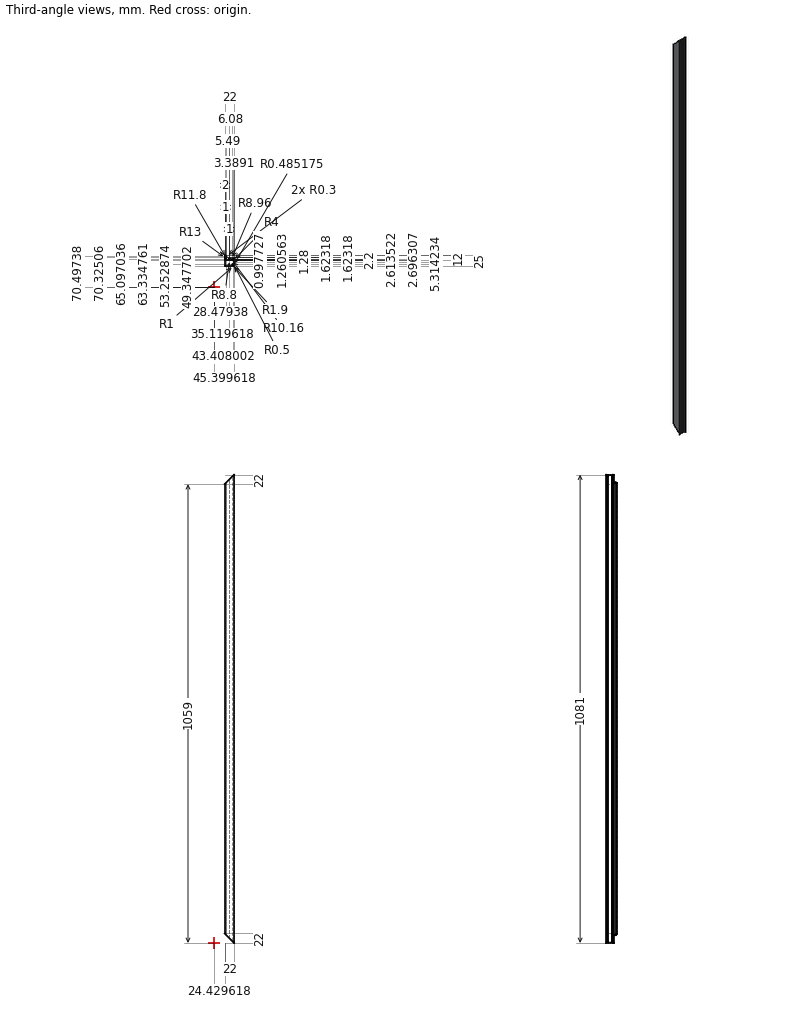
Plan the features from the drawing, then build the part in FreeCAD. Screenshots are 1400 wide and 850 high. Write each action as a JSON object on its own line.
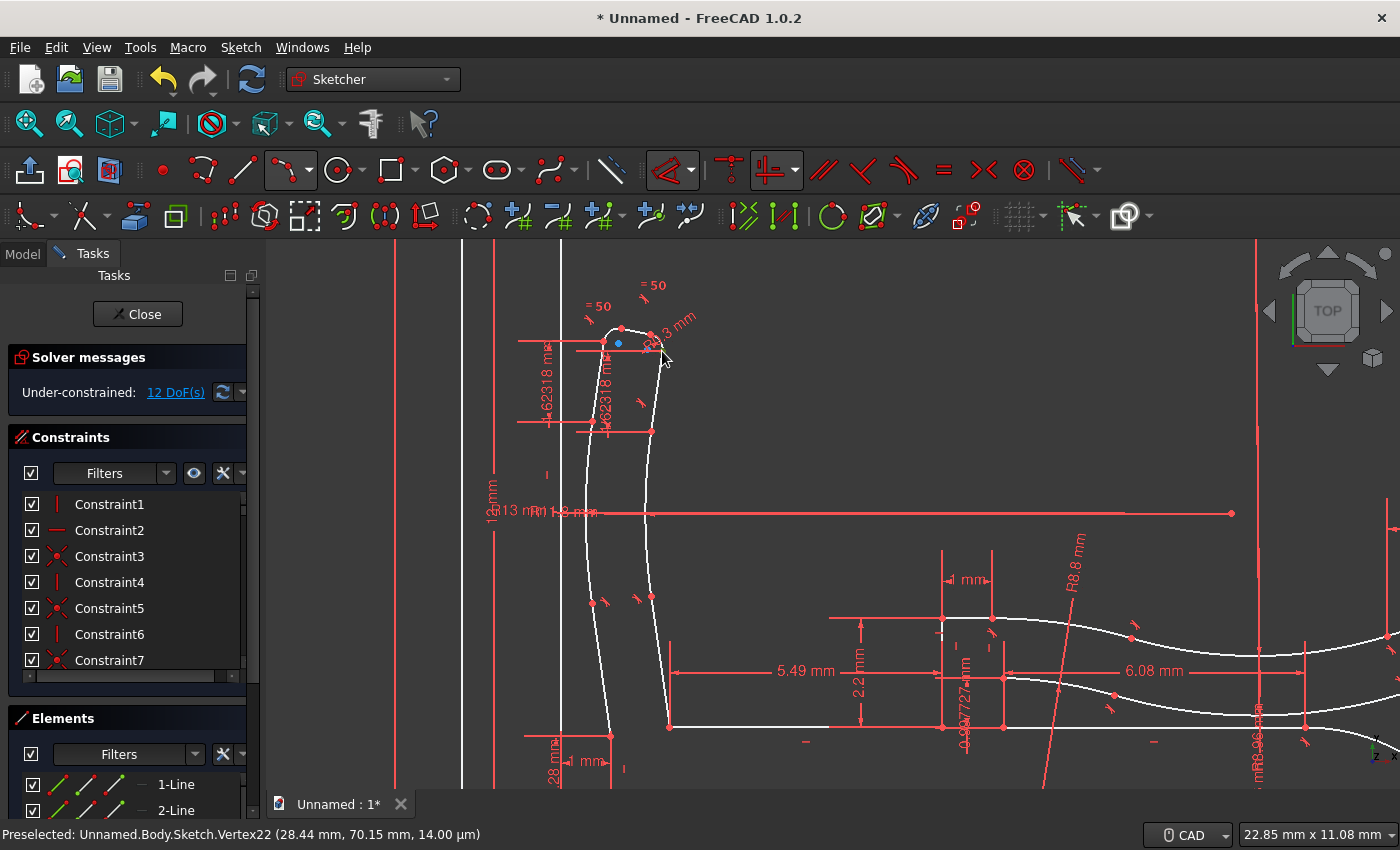
{"action": "left_click", "coordinate": [694, 170]}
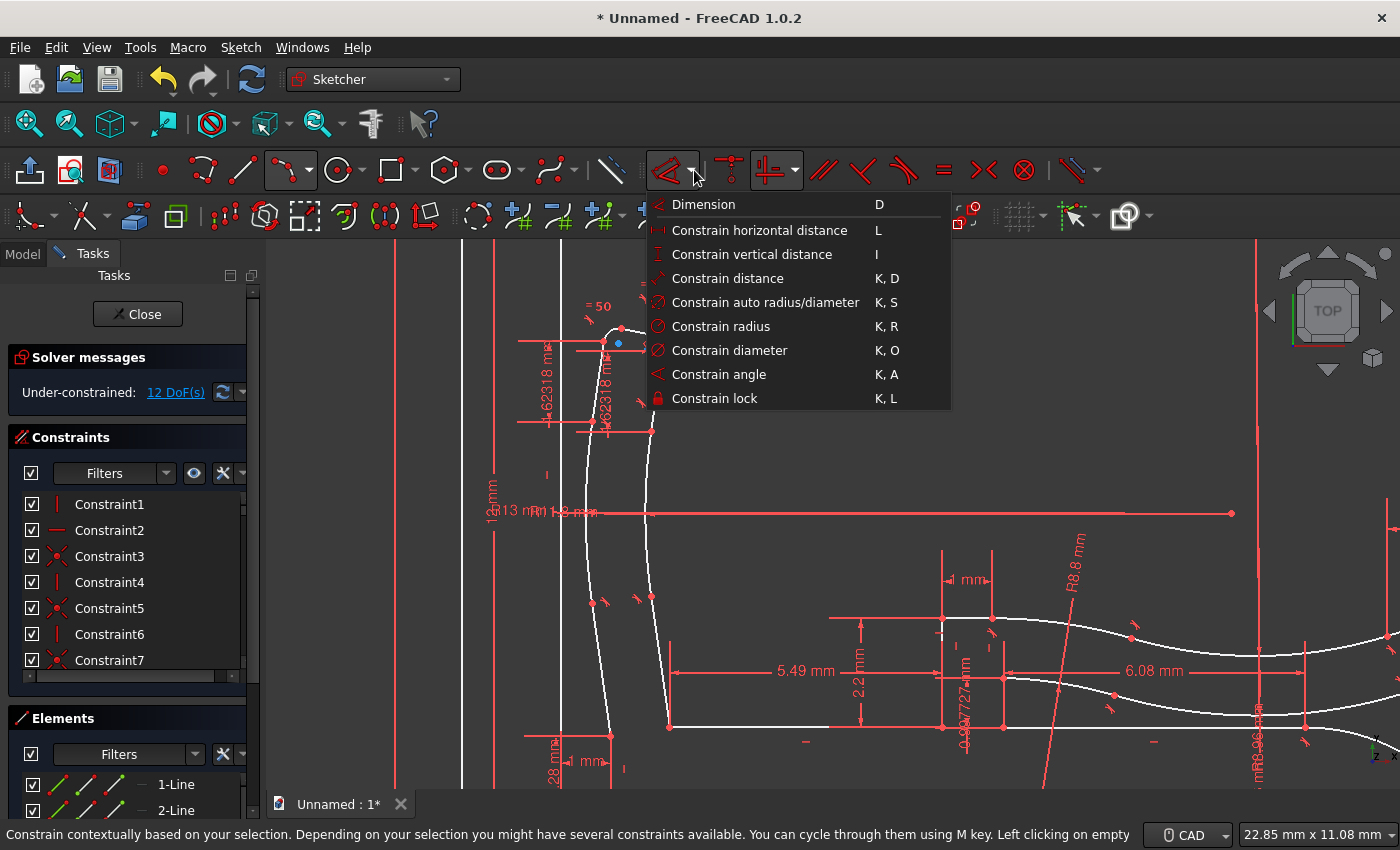
{"action": "left_click", "coordinate": [799, 230]}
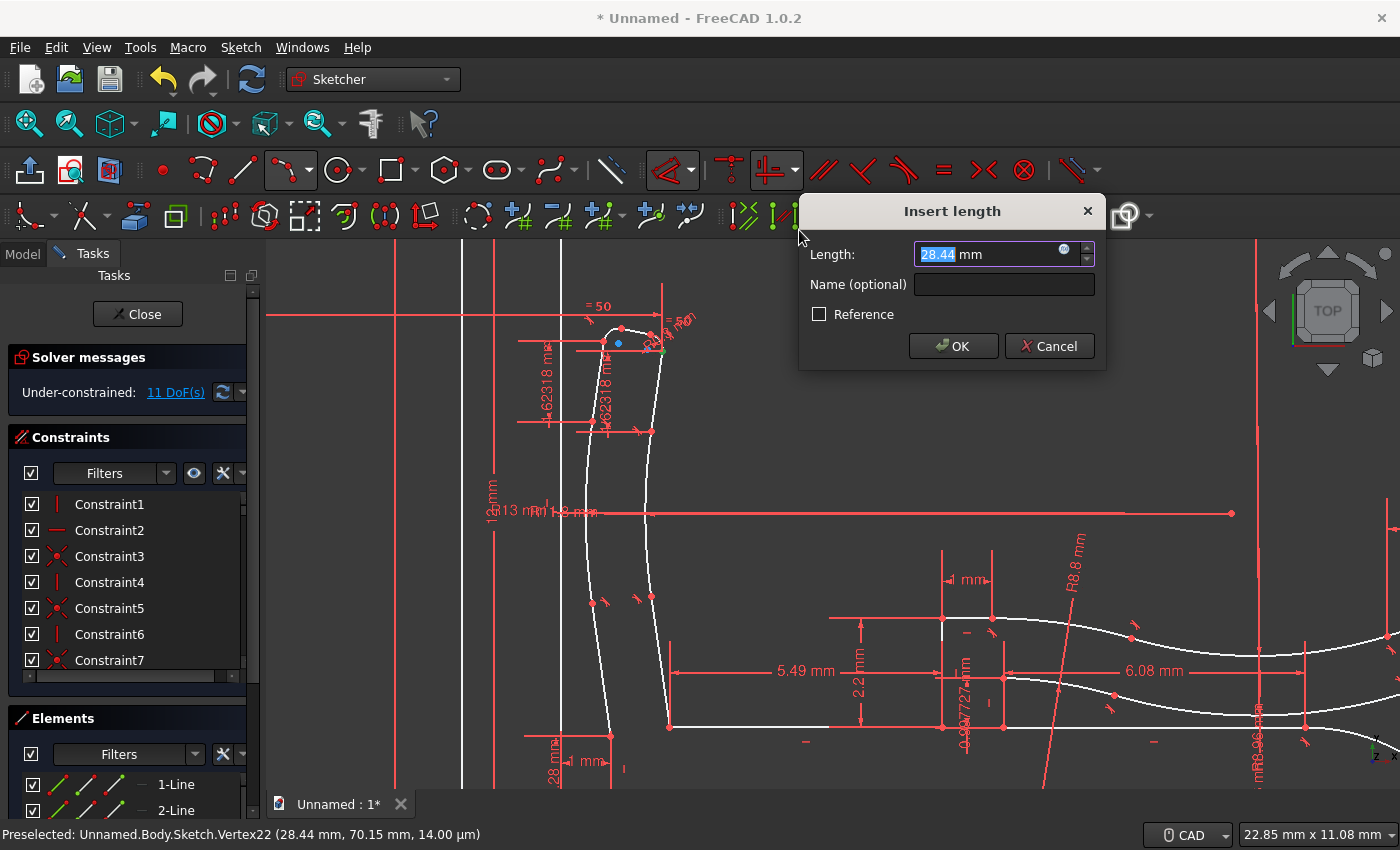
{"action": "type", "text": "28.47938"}
{"action": "key", "text": "Return"}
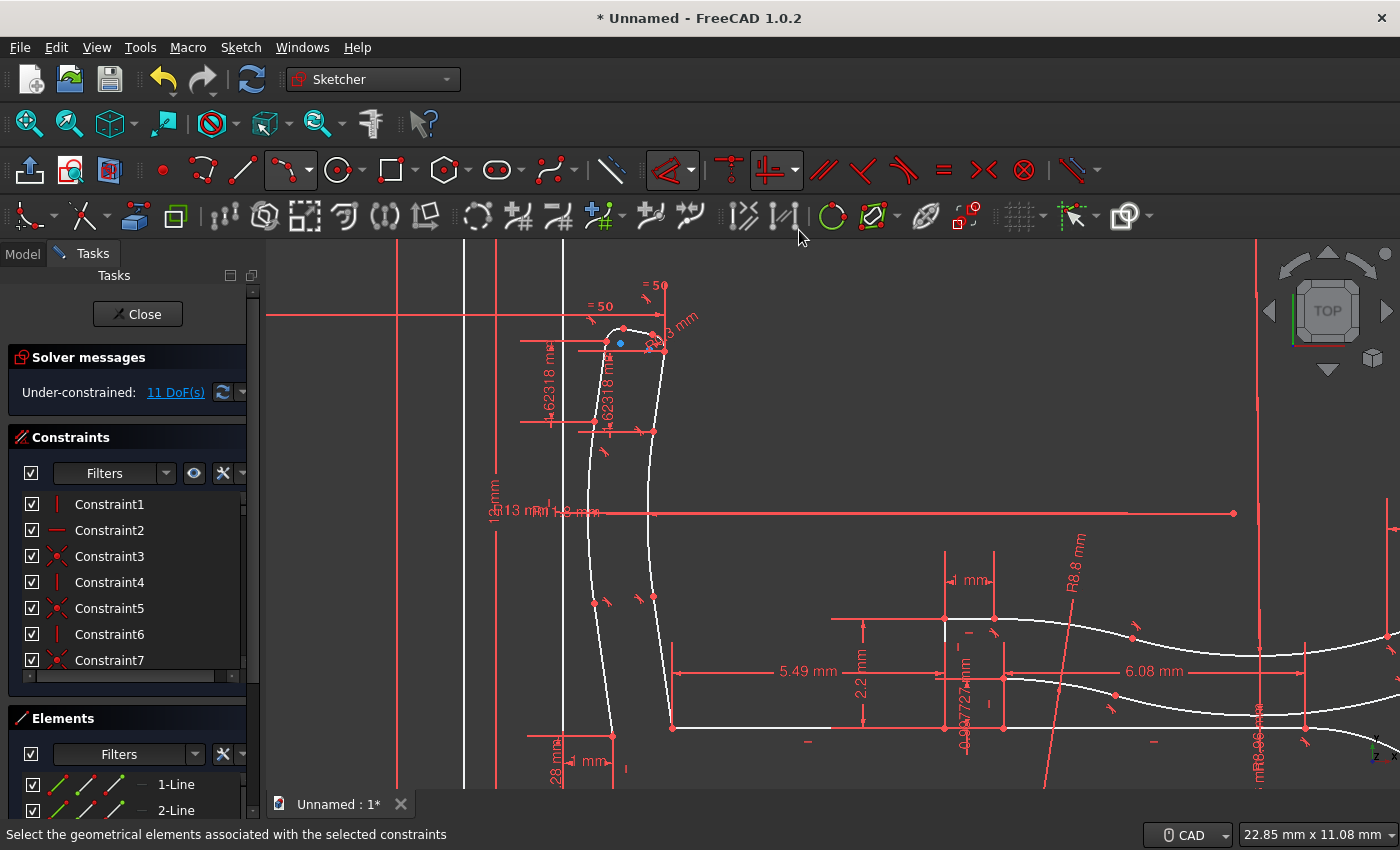
{"action": "left_click", "coordinate": [653, 335]}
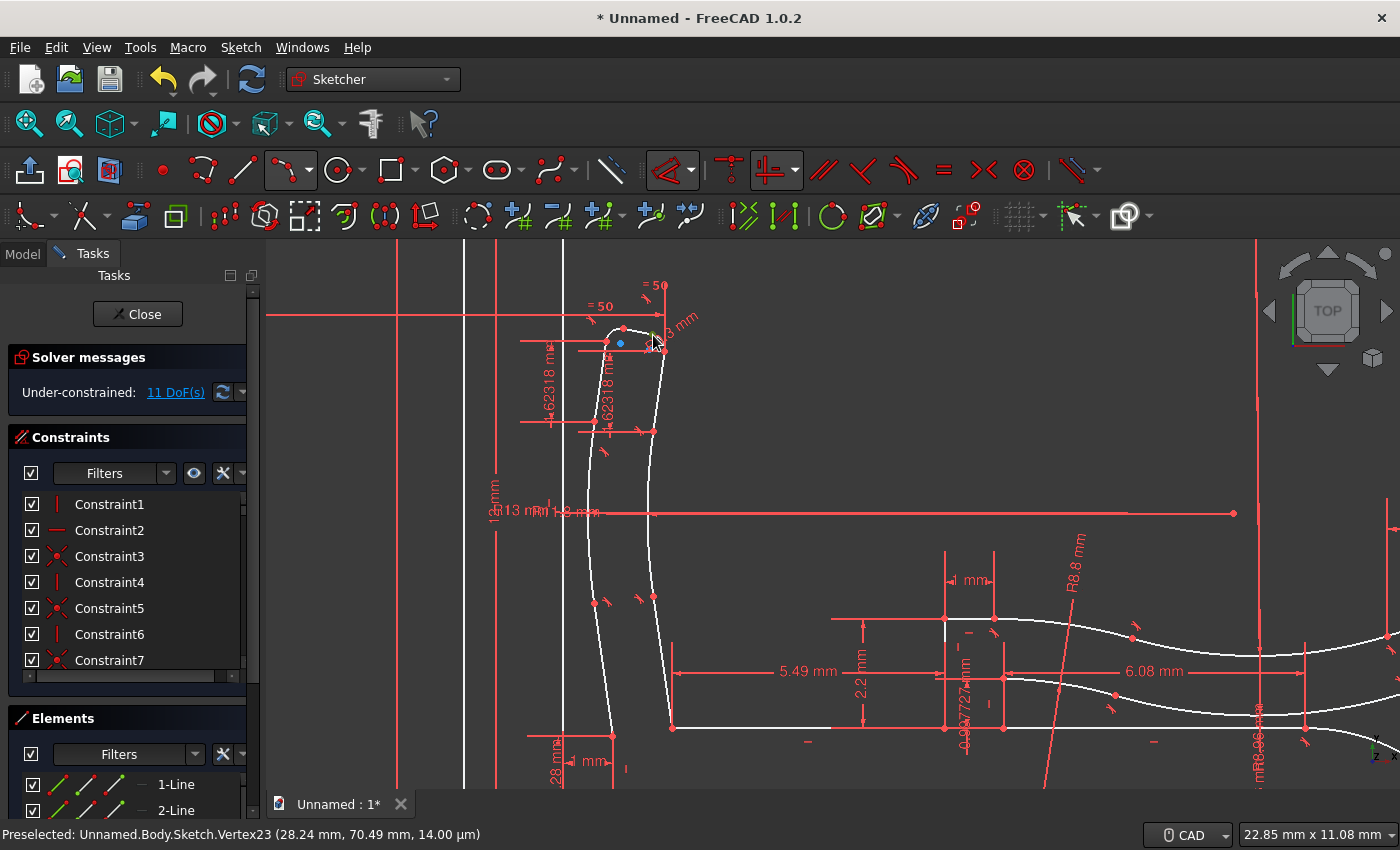
{"action": "key", "text": "i"}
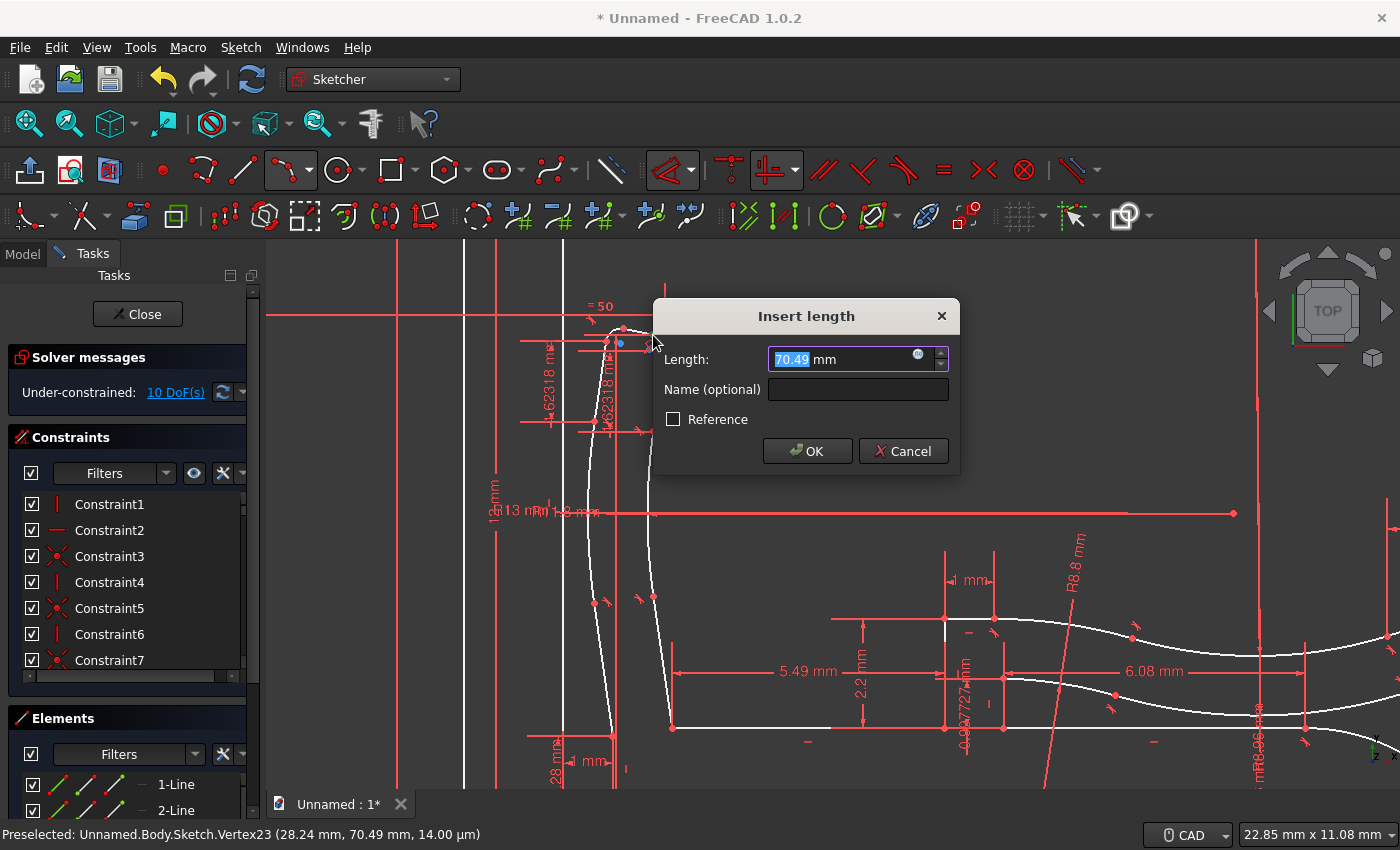
{"action": "type", "text": "70.49738"}
{"action": "key", "text": "Return"}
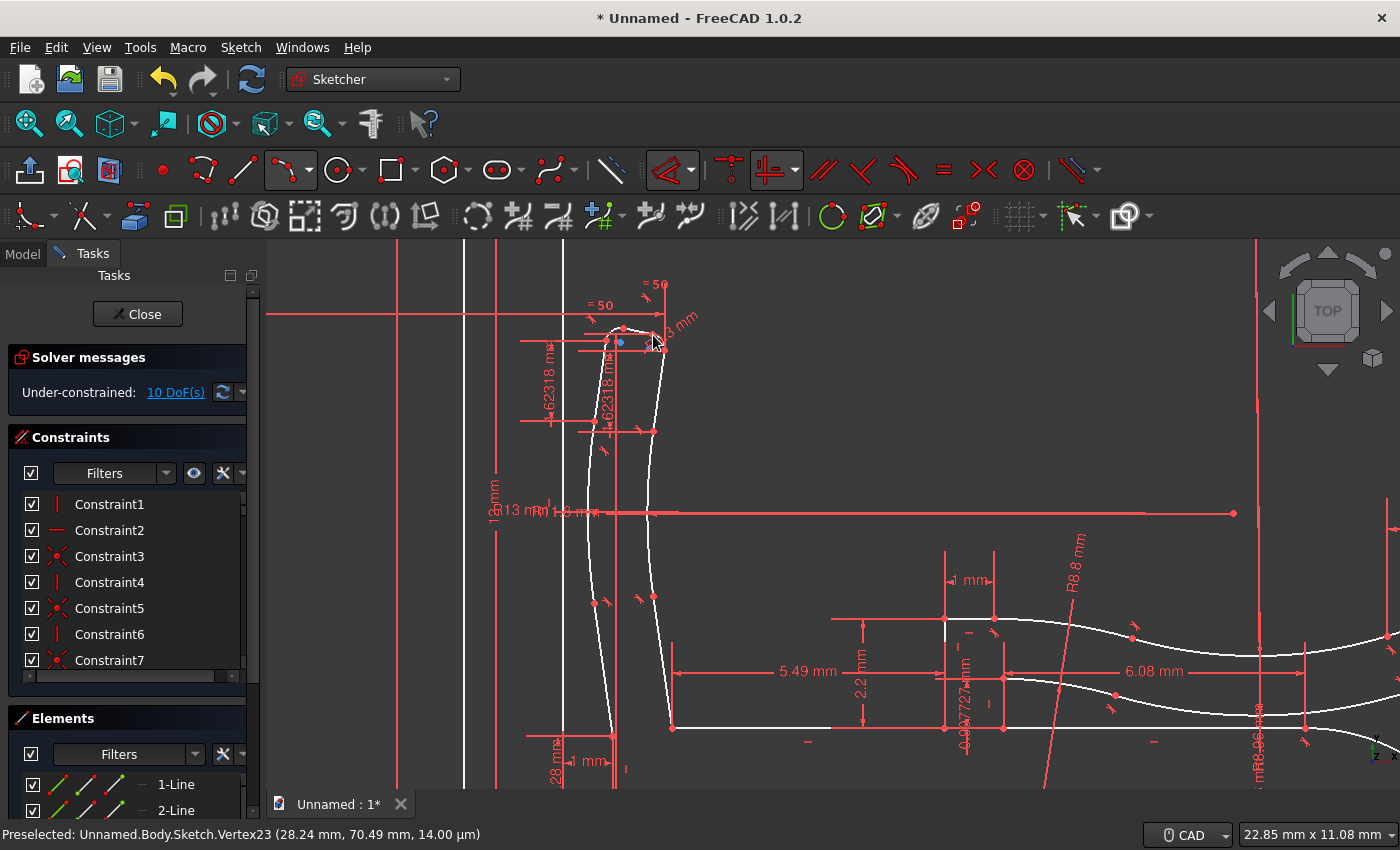
{"action": "left_click", "coordinate": [606, 341]}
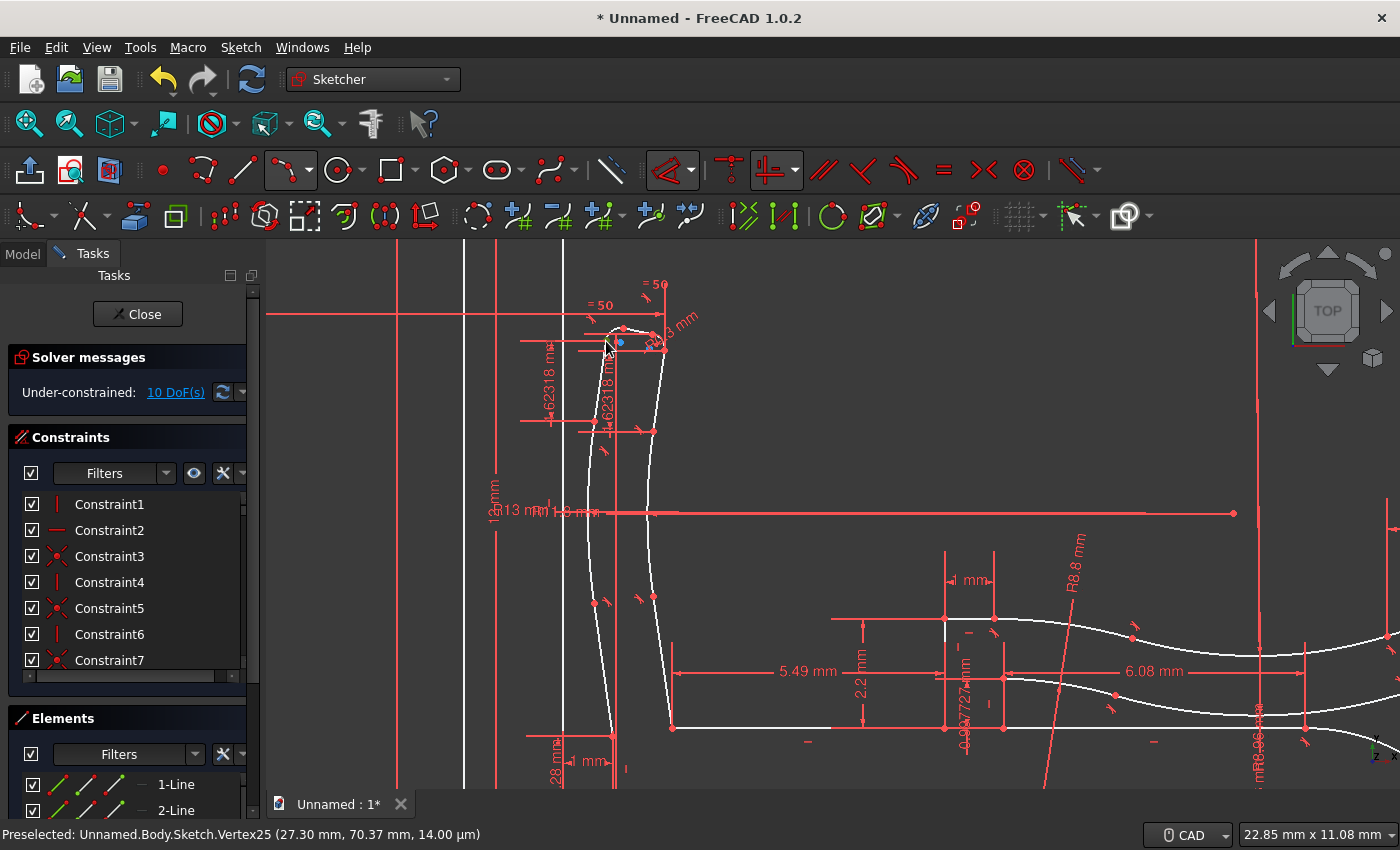
{"action": "key", "text": "i"}